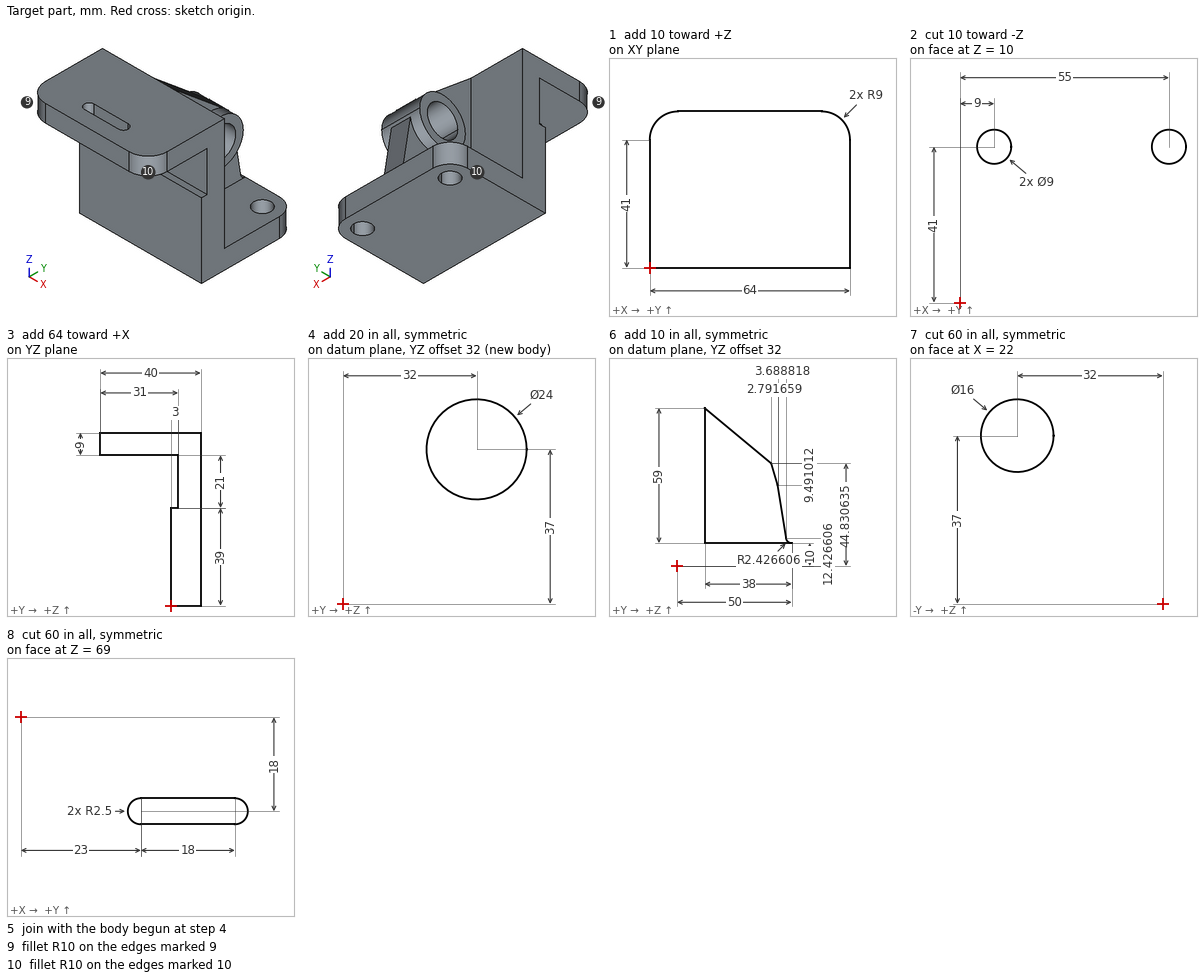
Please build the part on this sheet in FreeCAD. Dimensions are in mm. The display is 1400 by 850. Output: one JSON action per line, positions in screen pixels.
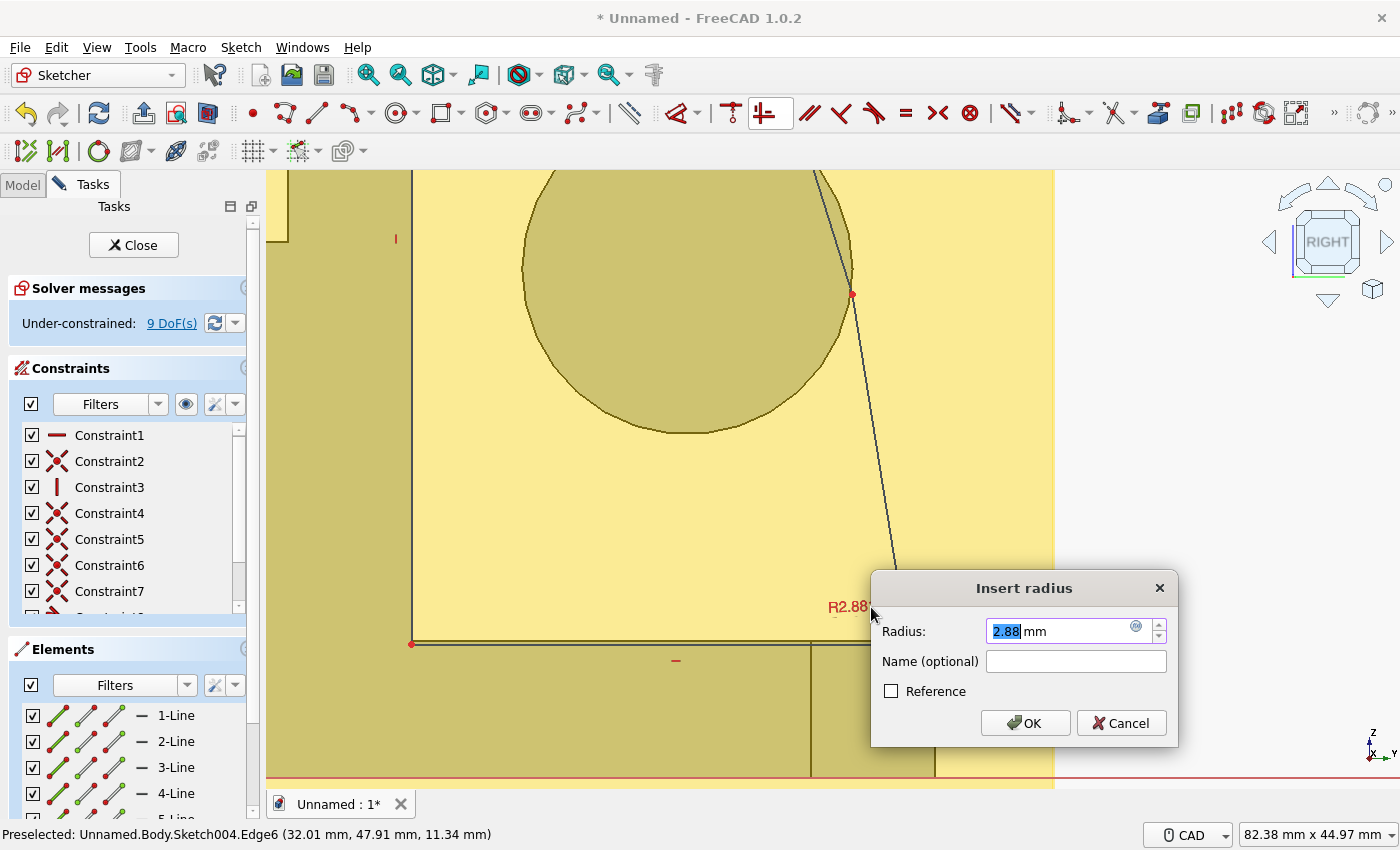
{"action": "type", "text": "2.426606"}
{"action": "key", "text": "Return"}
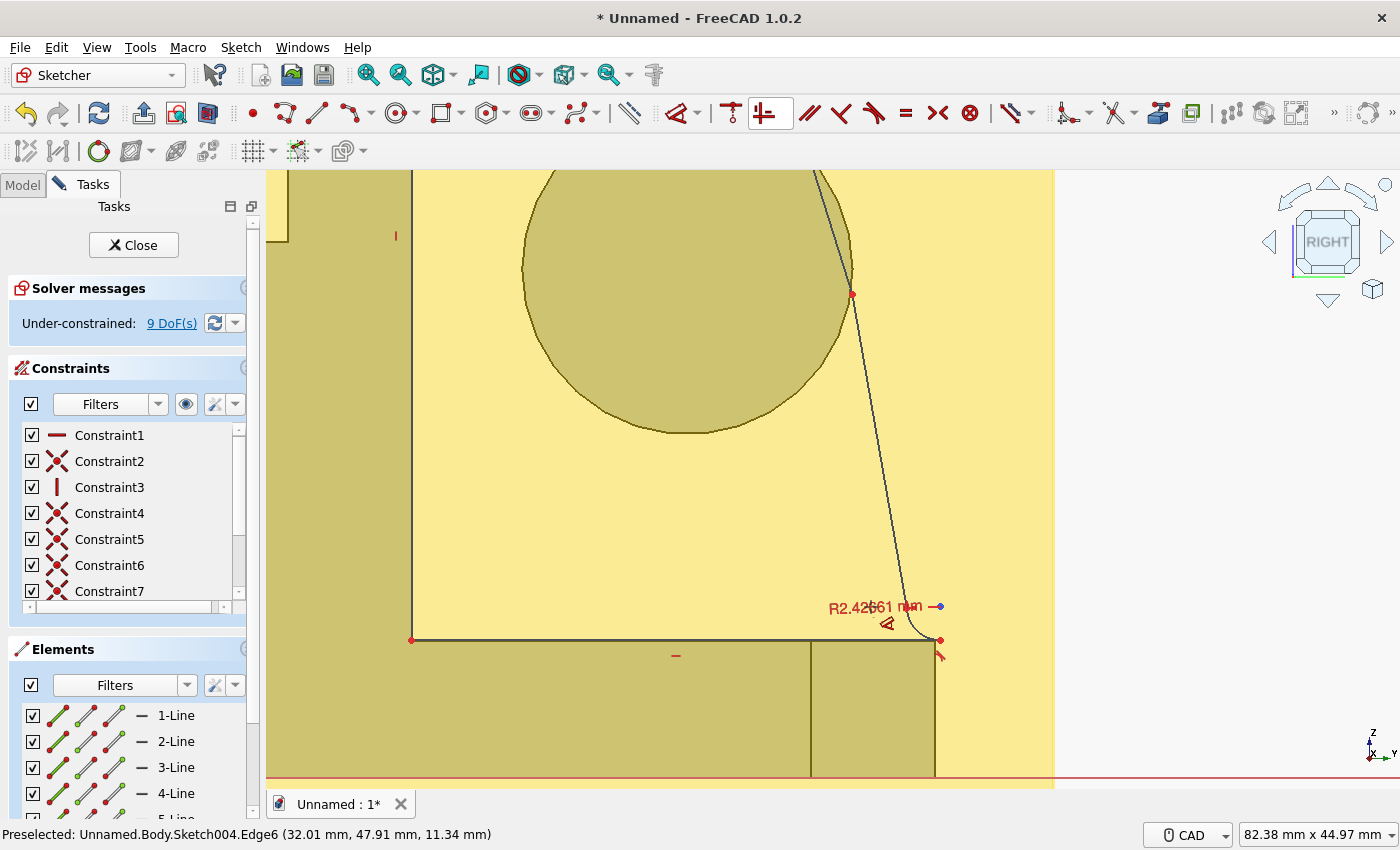
{"action": "left_click", "coordinate": [782, 640]}
{"action": "left_click", "coordinate": [676, 674]}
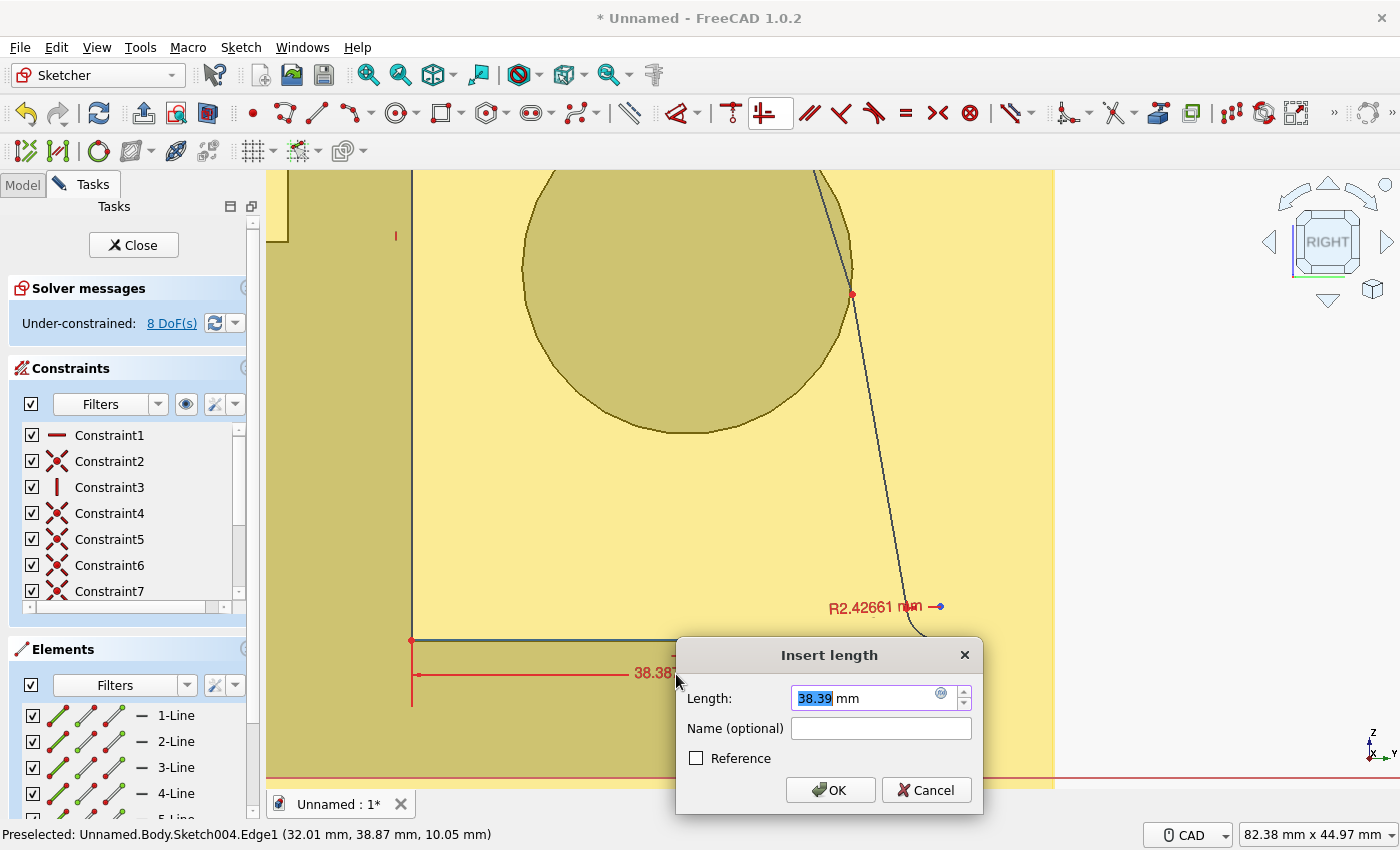
{"action": "type", "text": "38"}
{"action": "key", "text": "Return"}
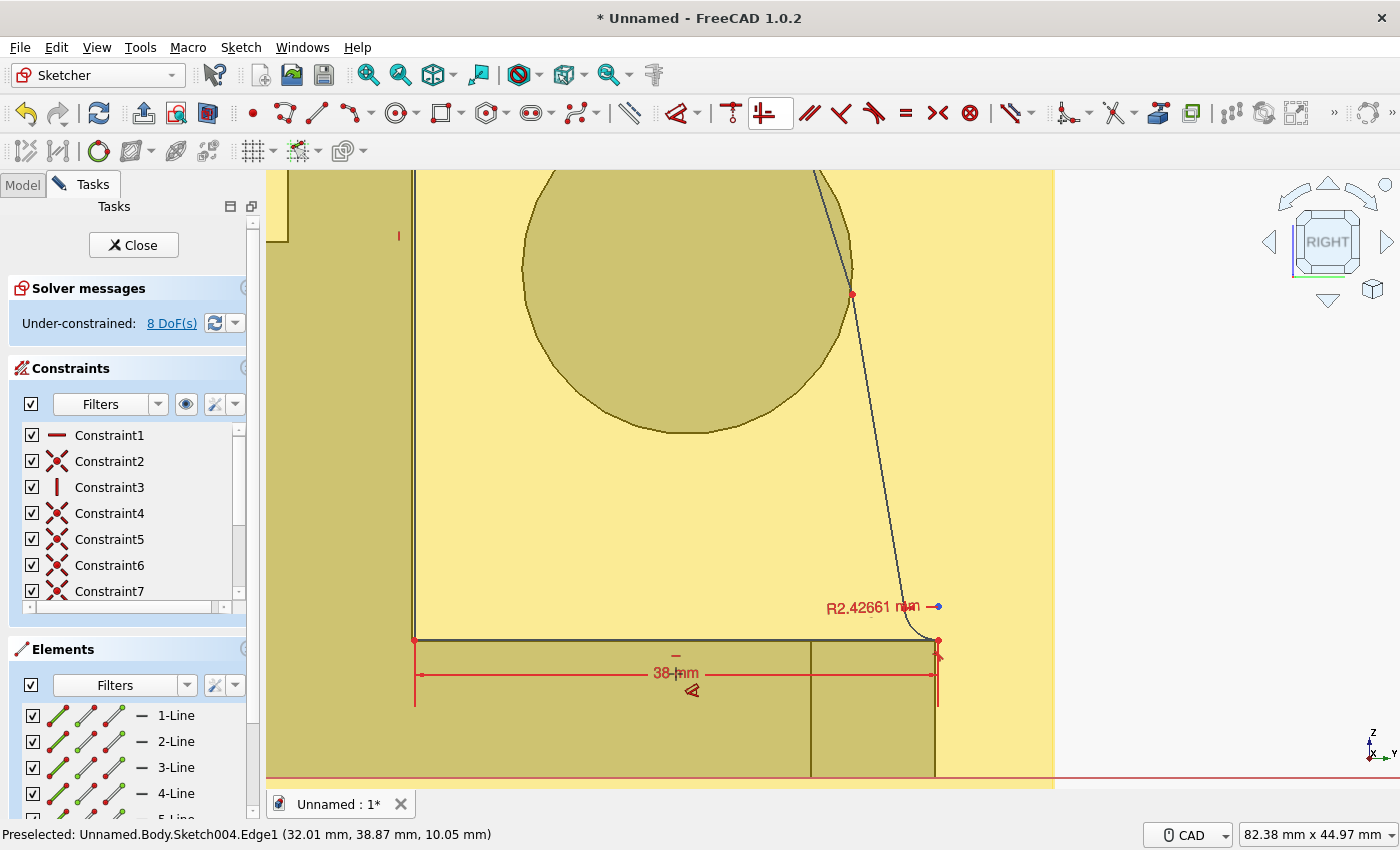
{"action": "left_click", "coordinate": [415, 398]}
{"action": "left_click", "coordinate": [381, 419]}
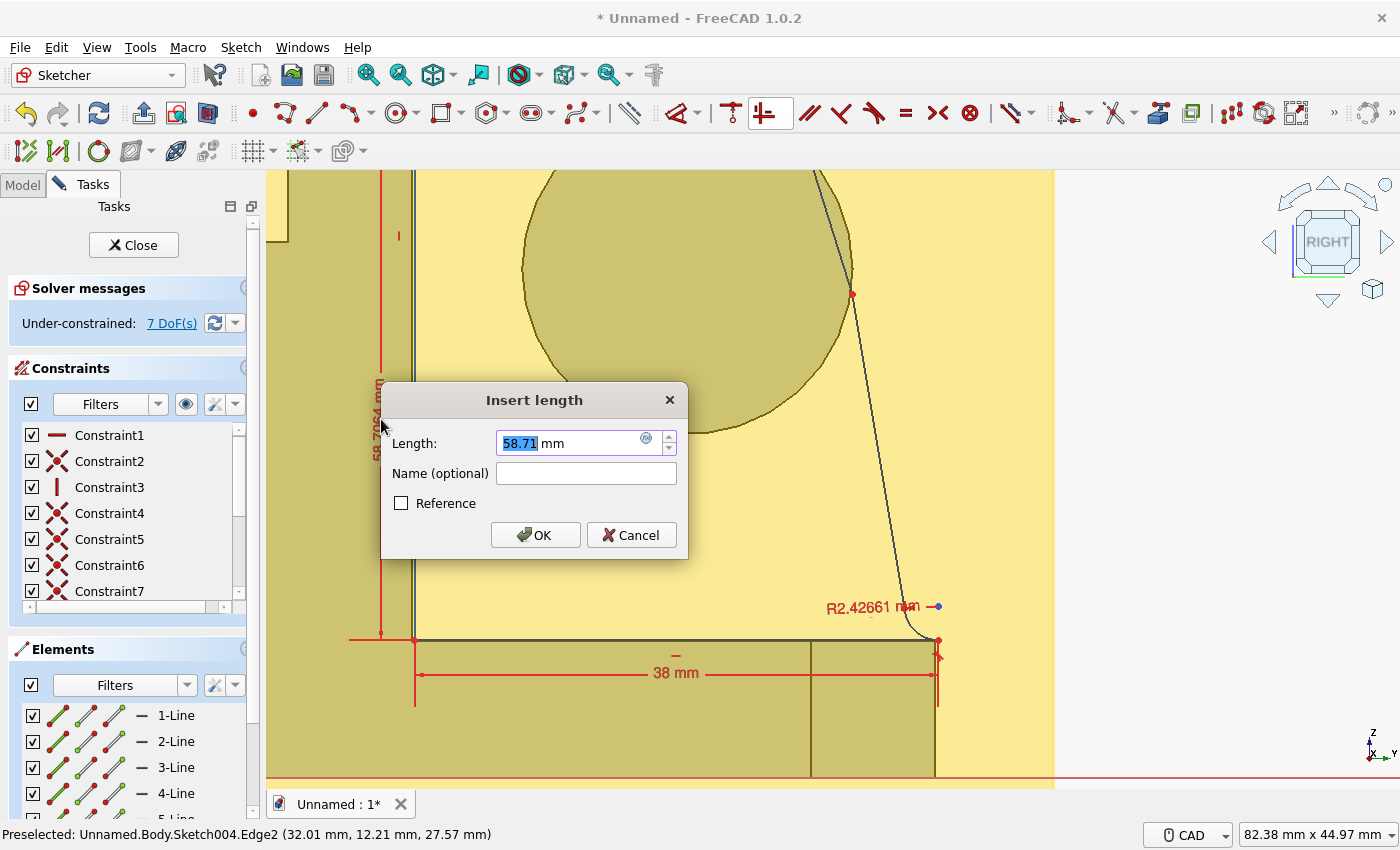
{"action": "type", "text": "59"}
{"action": "key", "text": "Return"}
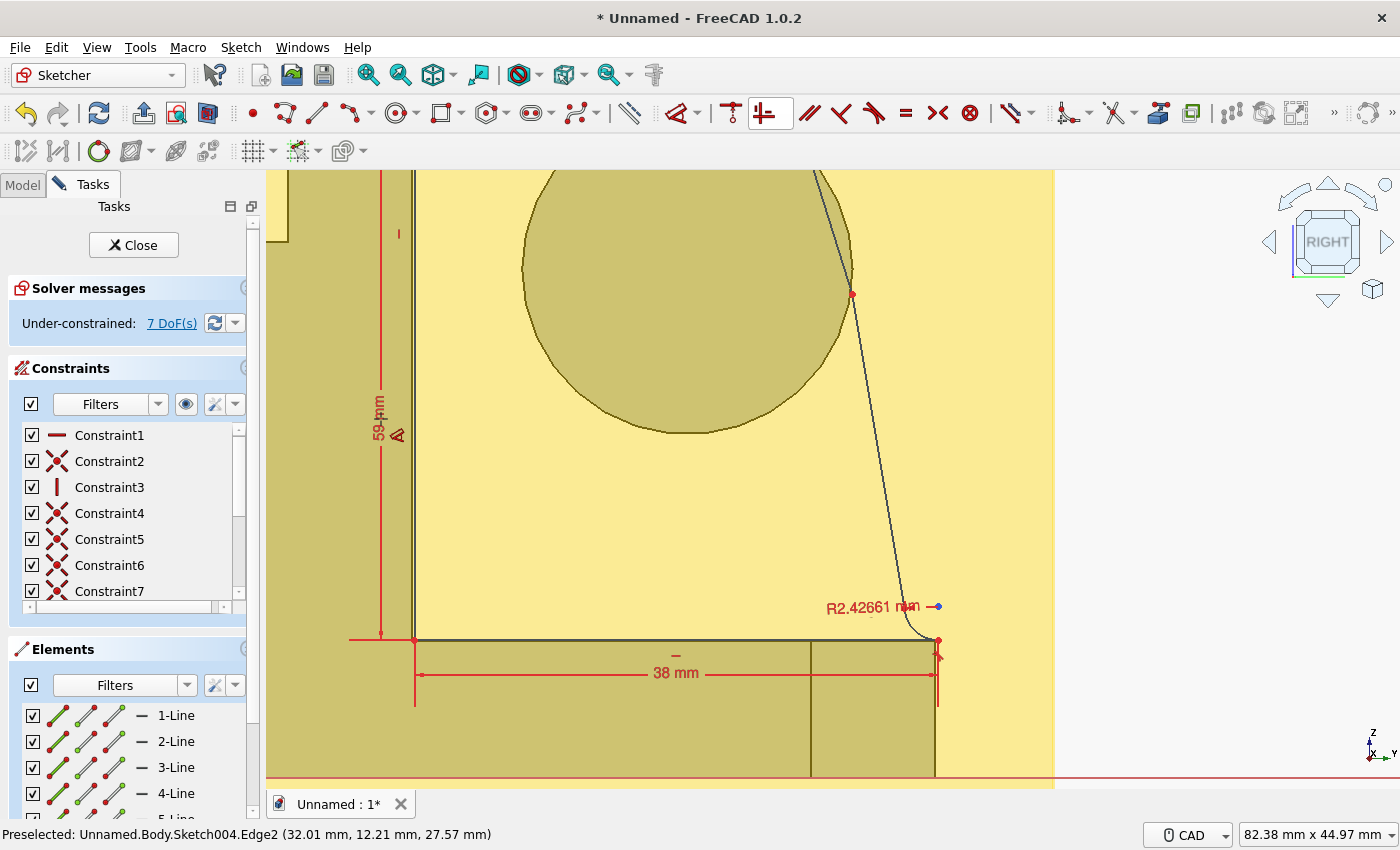
{"action": "left_click", "coordinate": [938, 640]}
{"action": "left_click", "coordinate": [616, 606]}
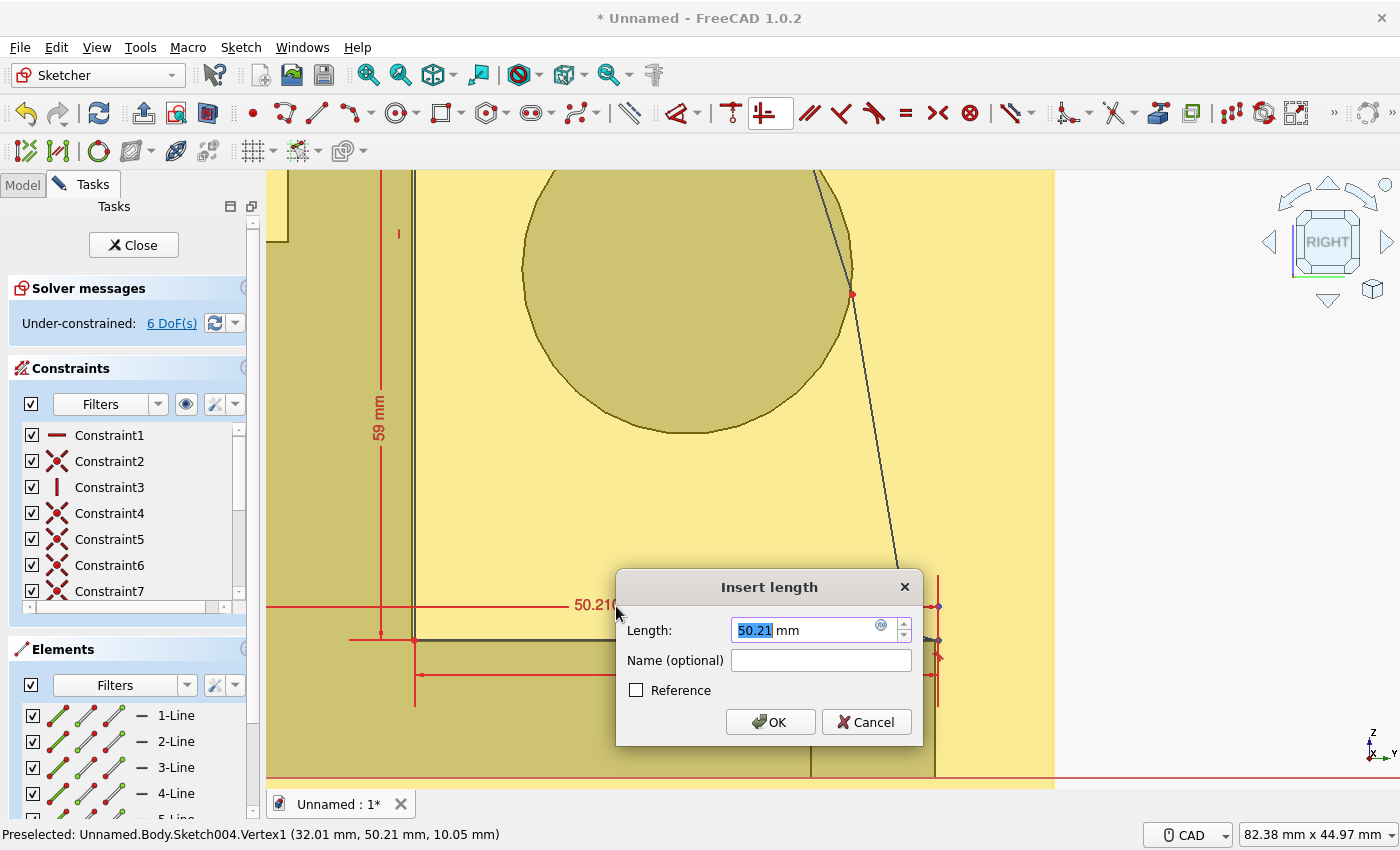
{"action": "type", "text": "50"}
{"action": "key", "text": "Return"}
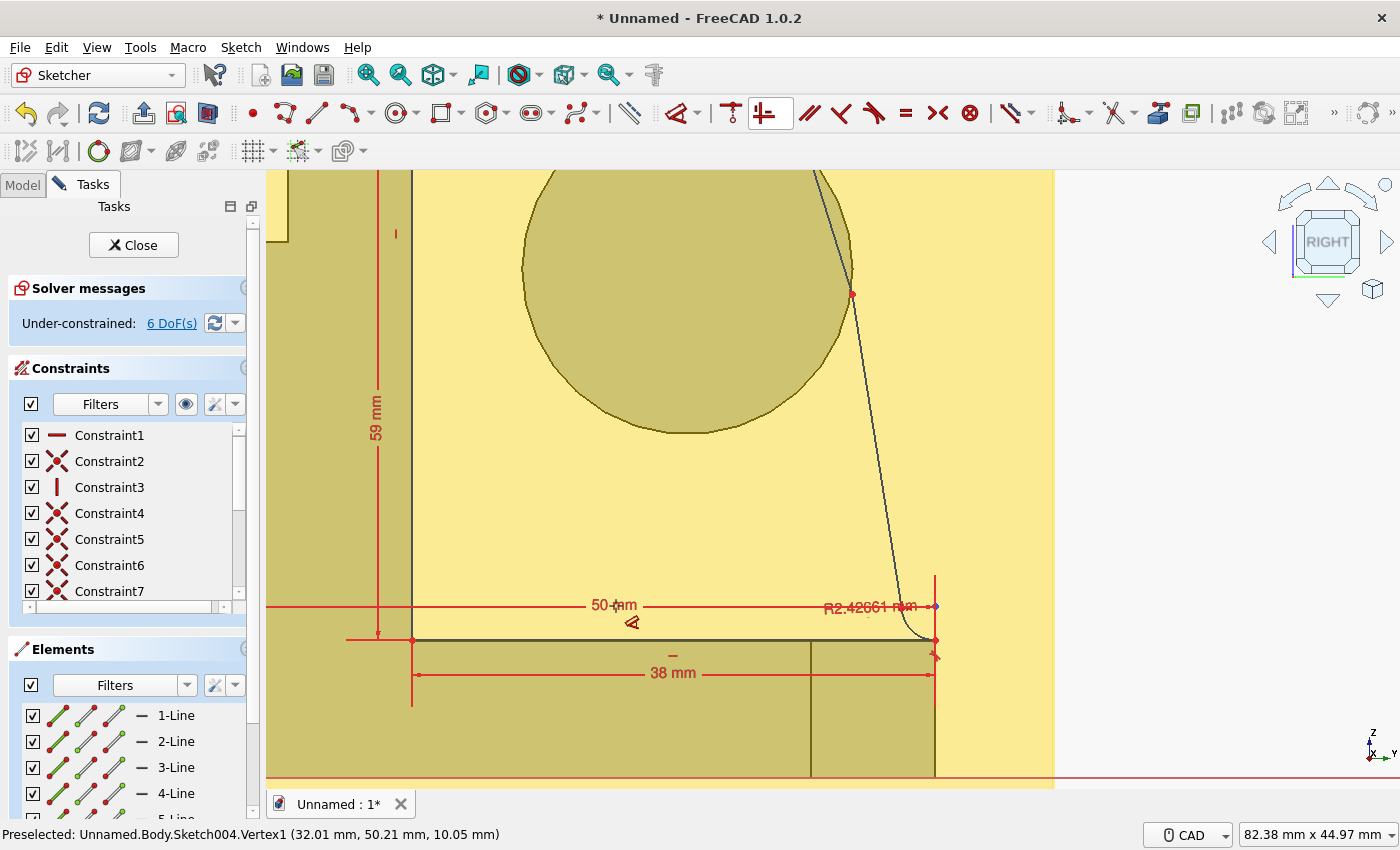
{"action": "left_click", "coordinate": [935, 640]}
{"action": "left_click", "coordinate": [969, 701]}